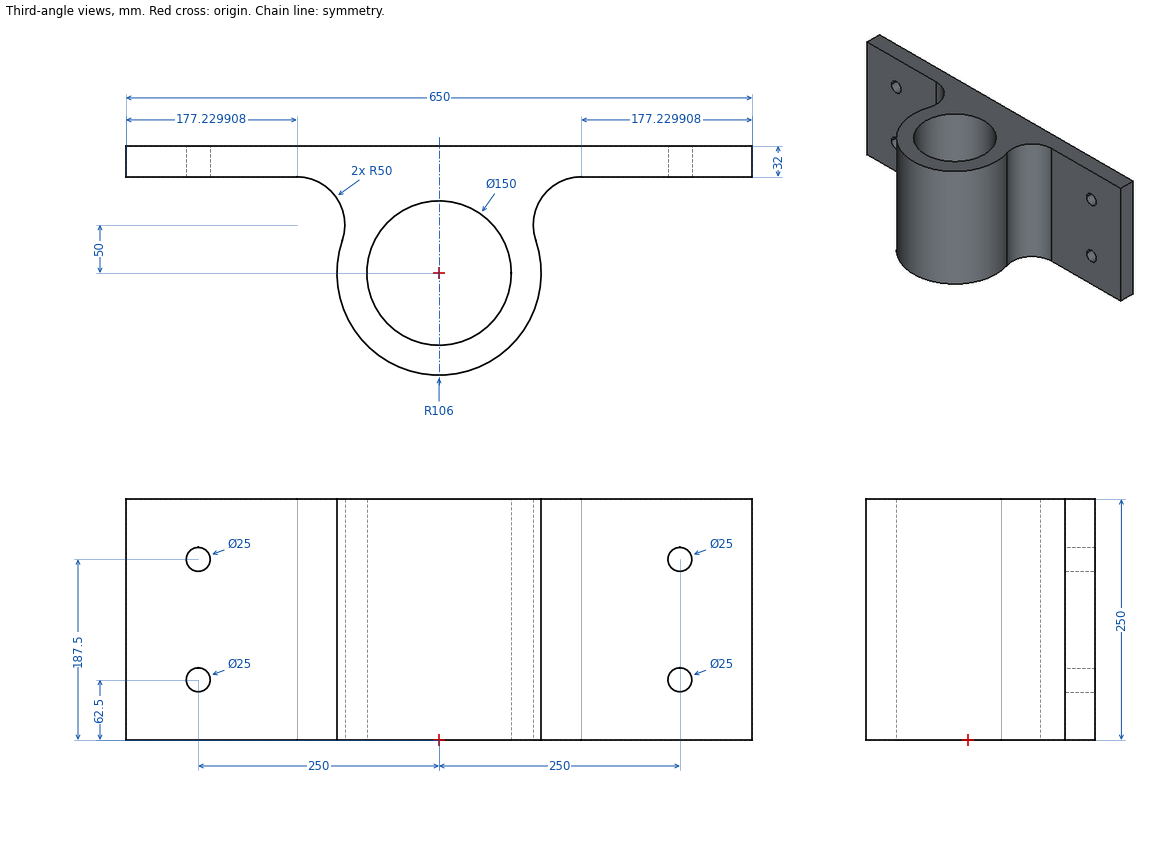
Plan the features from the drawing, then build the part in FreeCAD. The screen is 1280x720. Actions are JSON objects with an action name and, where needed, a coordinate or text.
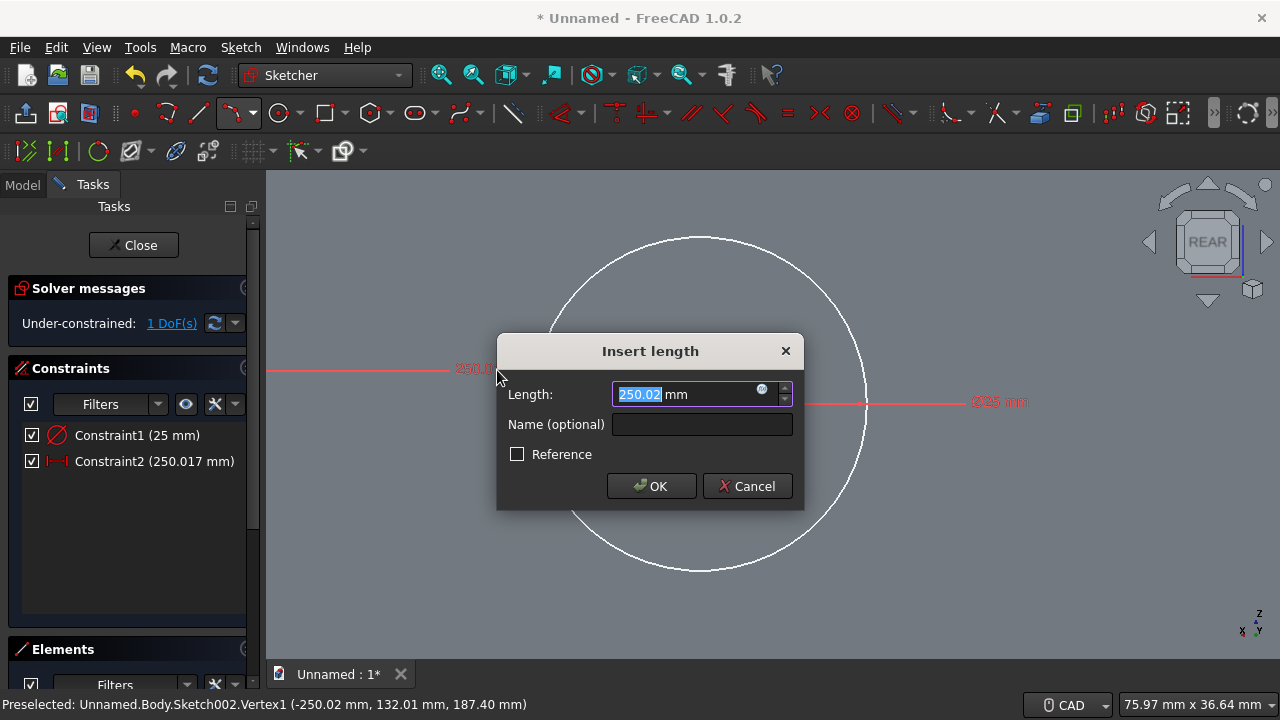
{"action": "type", "text": "250"}
{"action": "key", "text": "Return"}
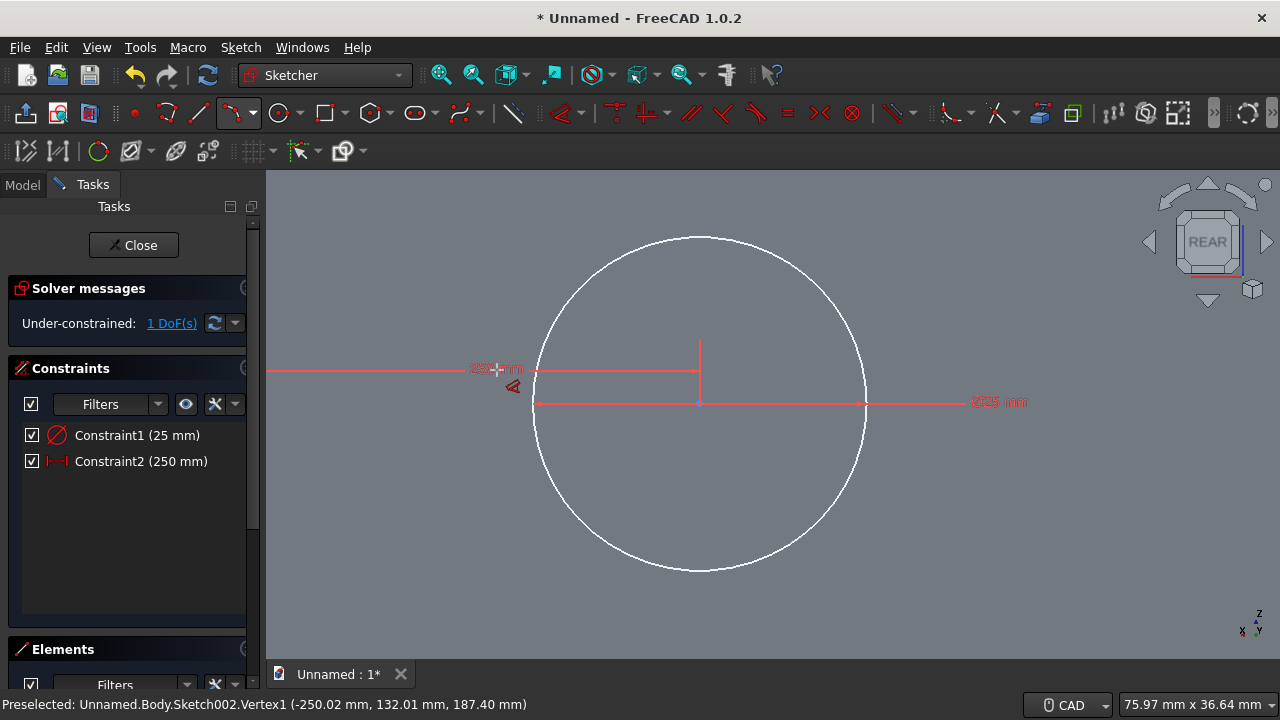
{"action": "left_click", "coordinate": [700, 404]}
{"action": "left_click", "coordinate": [734, 518]}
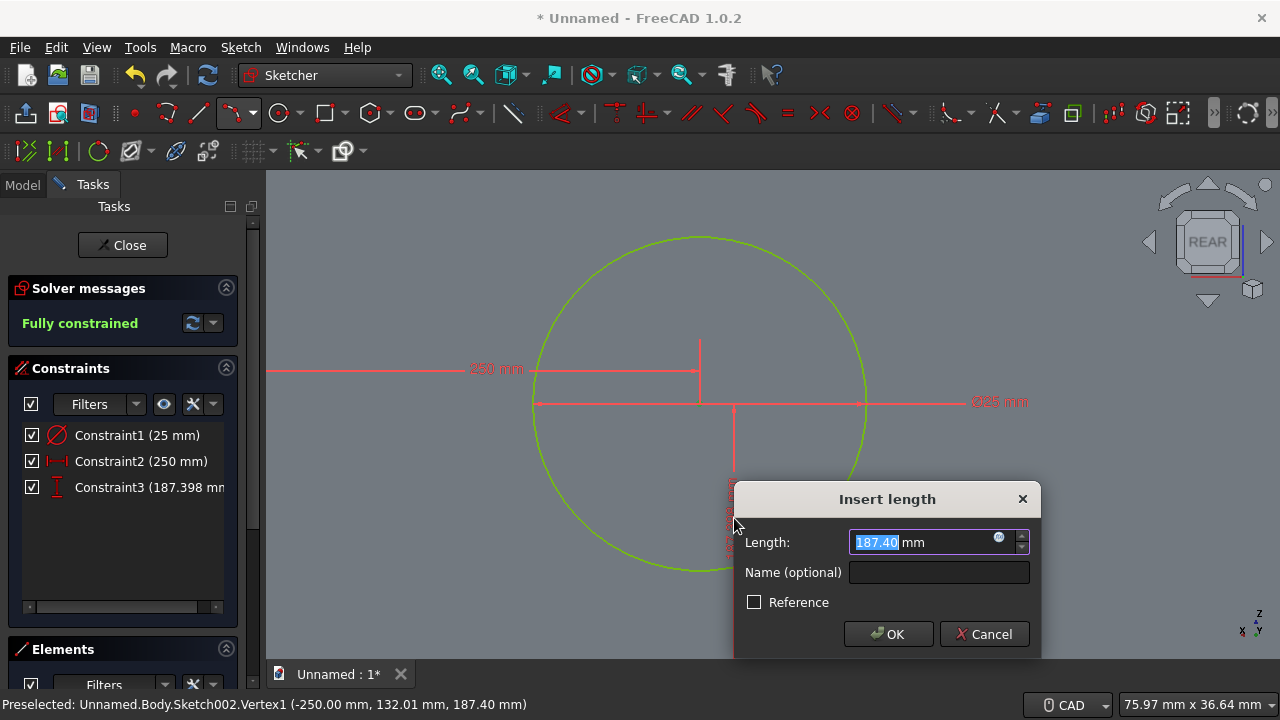
{"action": "type", "text": "187.5"}
{"action": "key", "text": "Return"}
{"action": "key", "text": "Escape"}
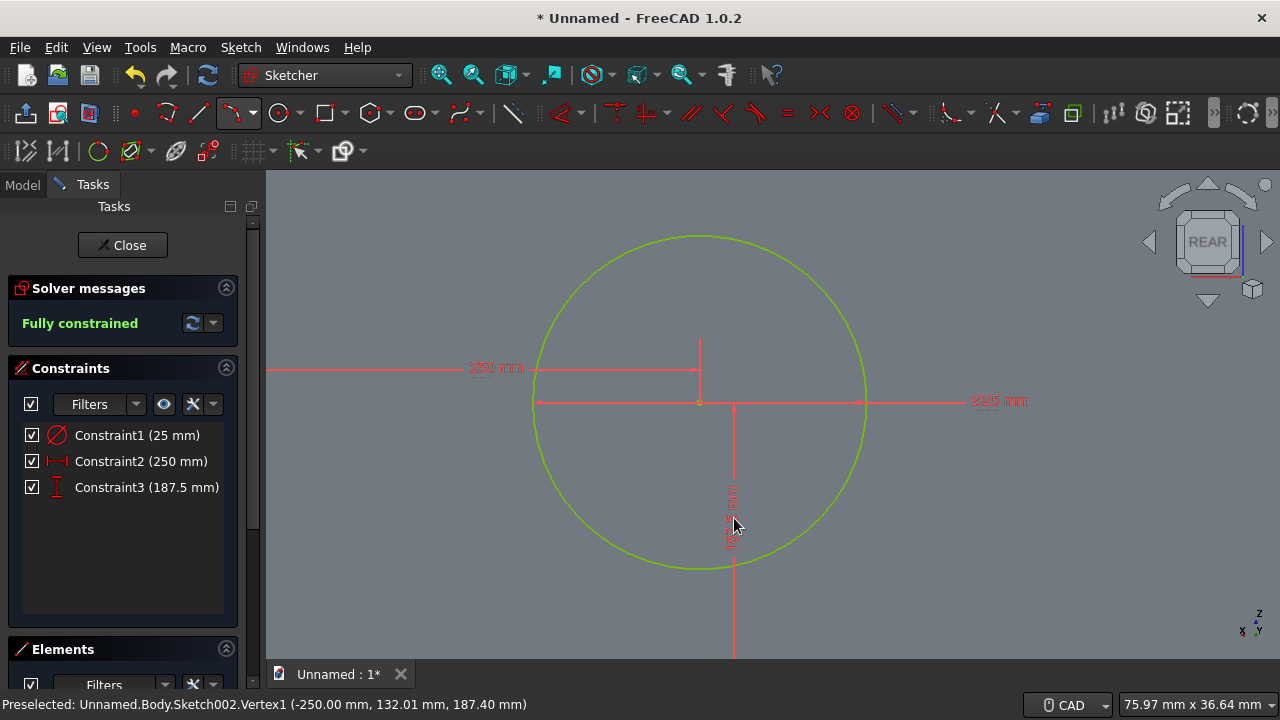
{"action": "left_click", "coordinate": [123, 245]}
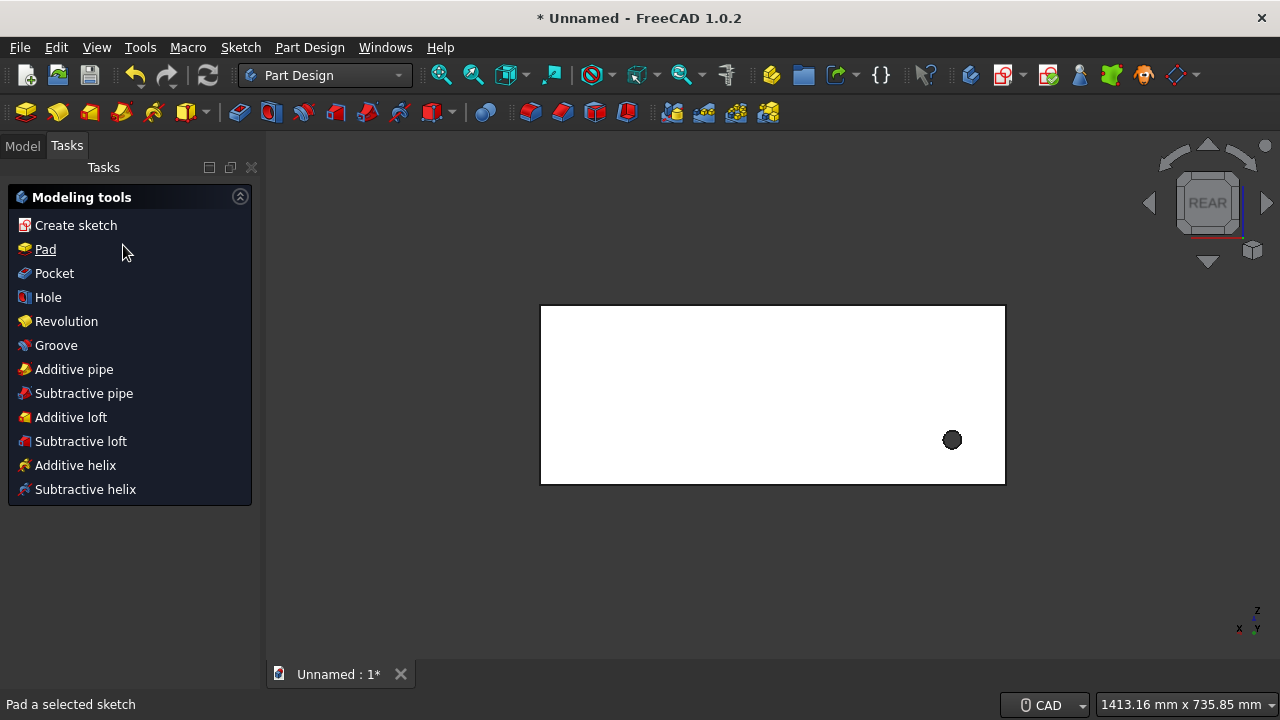
{"action": "left_click", "coordinate": [240, 112]}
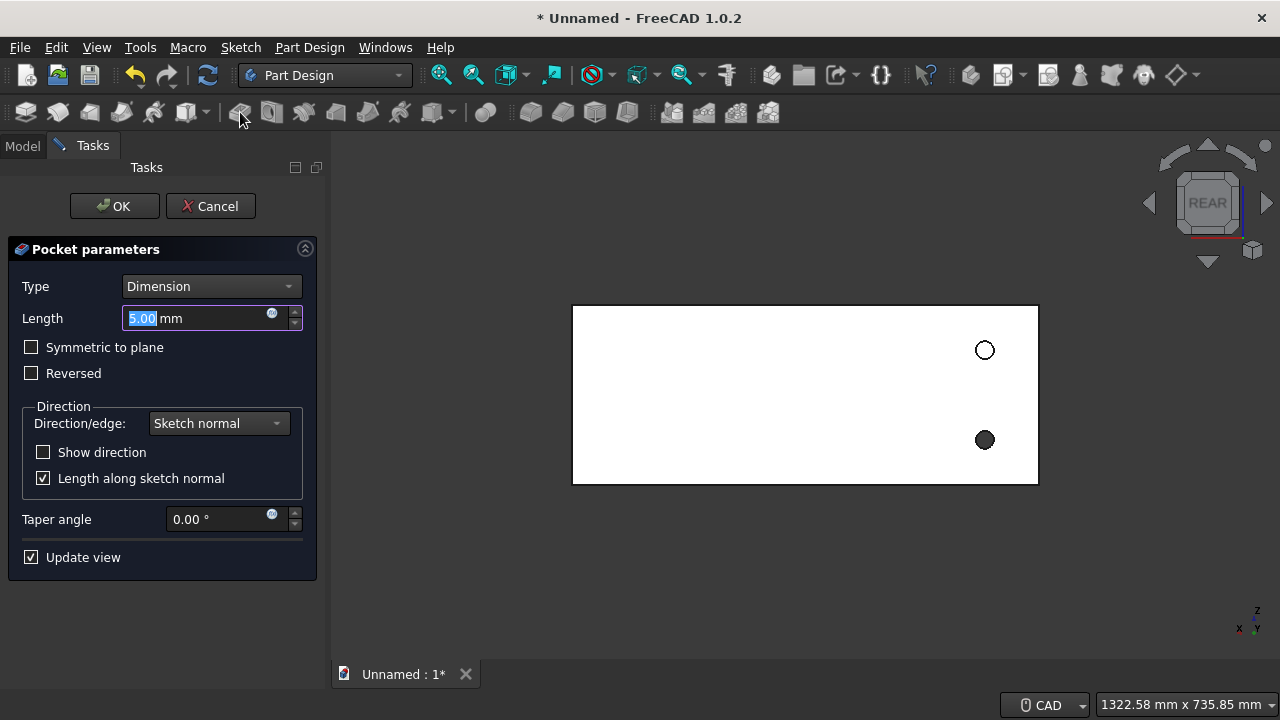
{"action": "left_click", "coordinate": [212, 286]}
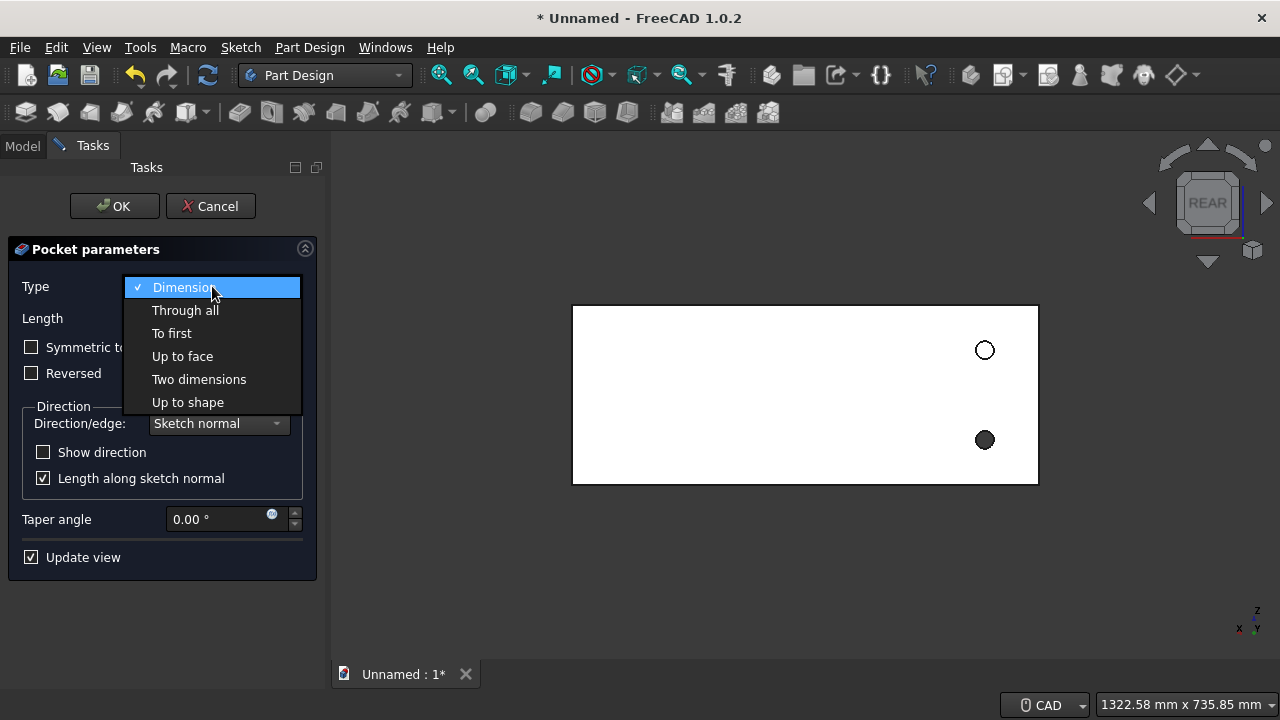
{"action": "left_click", "coordinate": [212, 334]}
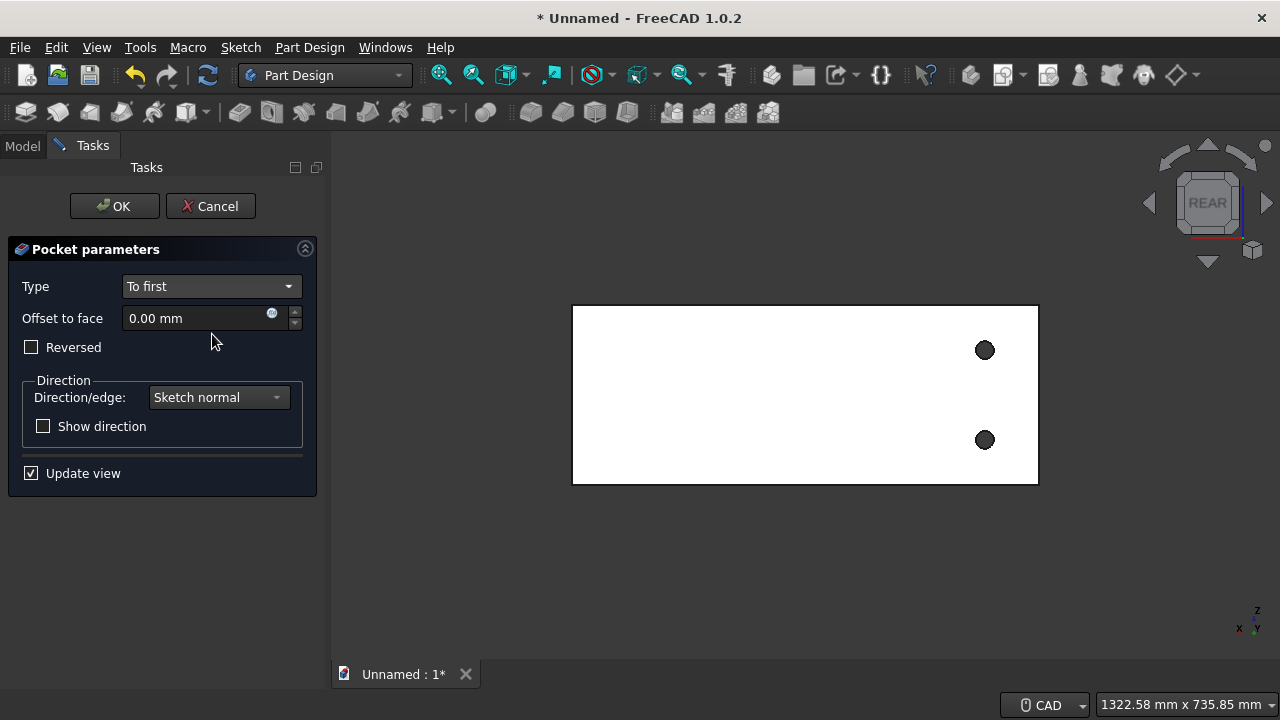
{"action": "left_click", "coordinate": [115, 206]}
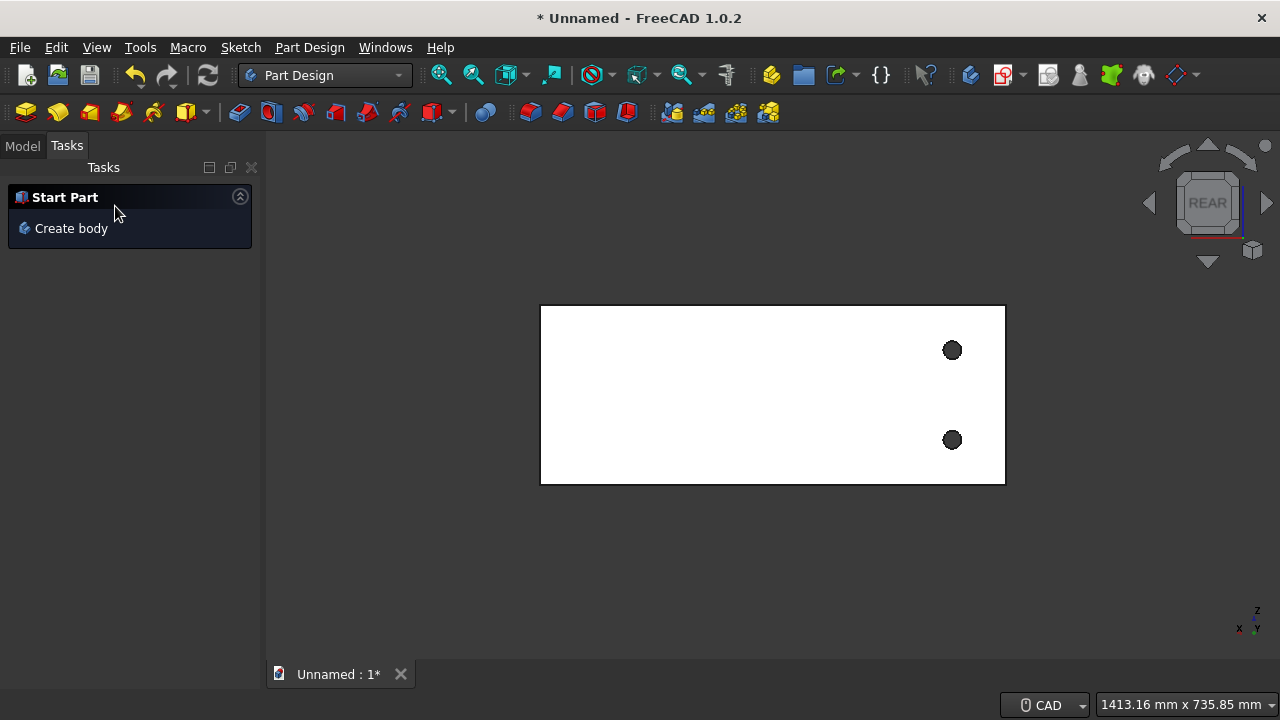
{"action": "left_click", "coordinate": [640, 394]}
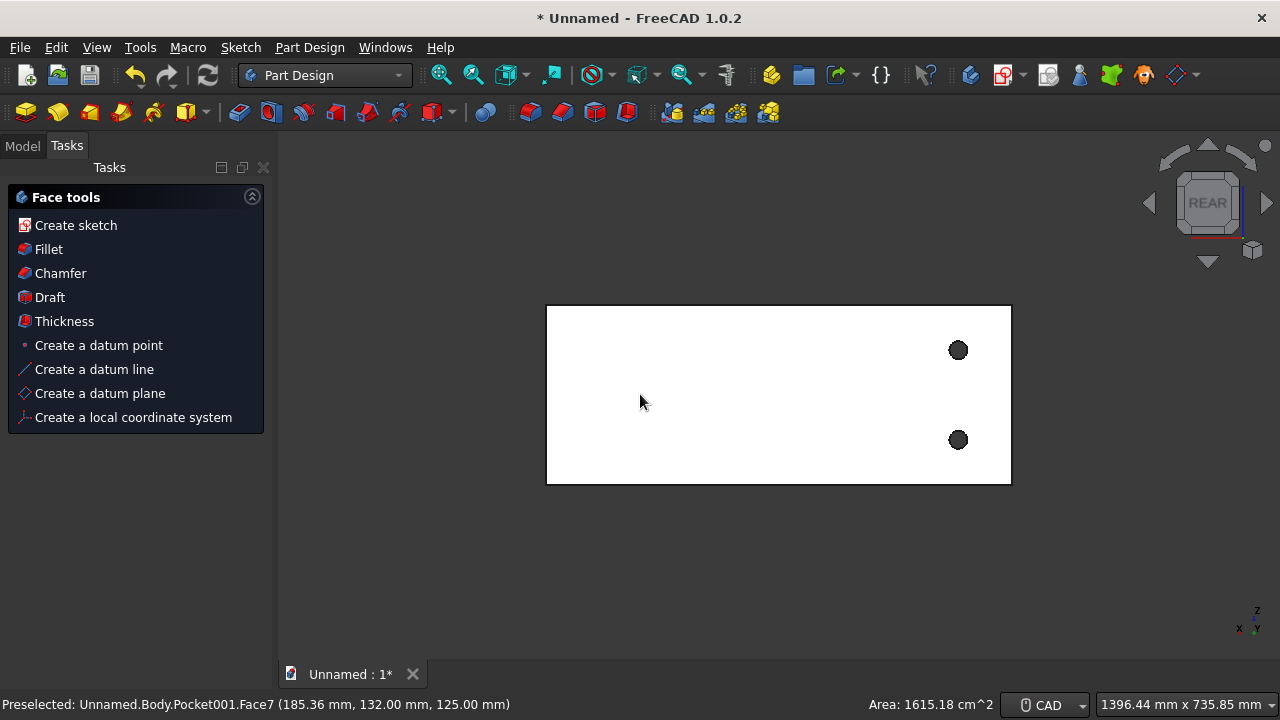
{"action": "left_click", "coordinate": [1004, 76]}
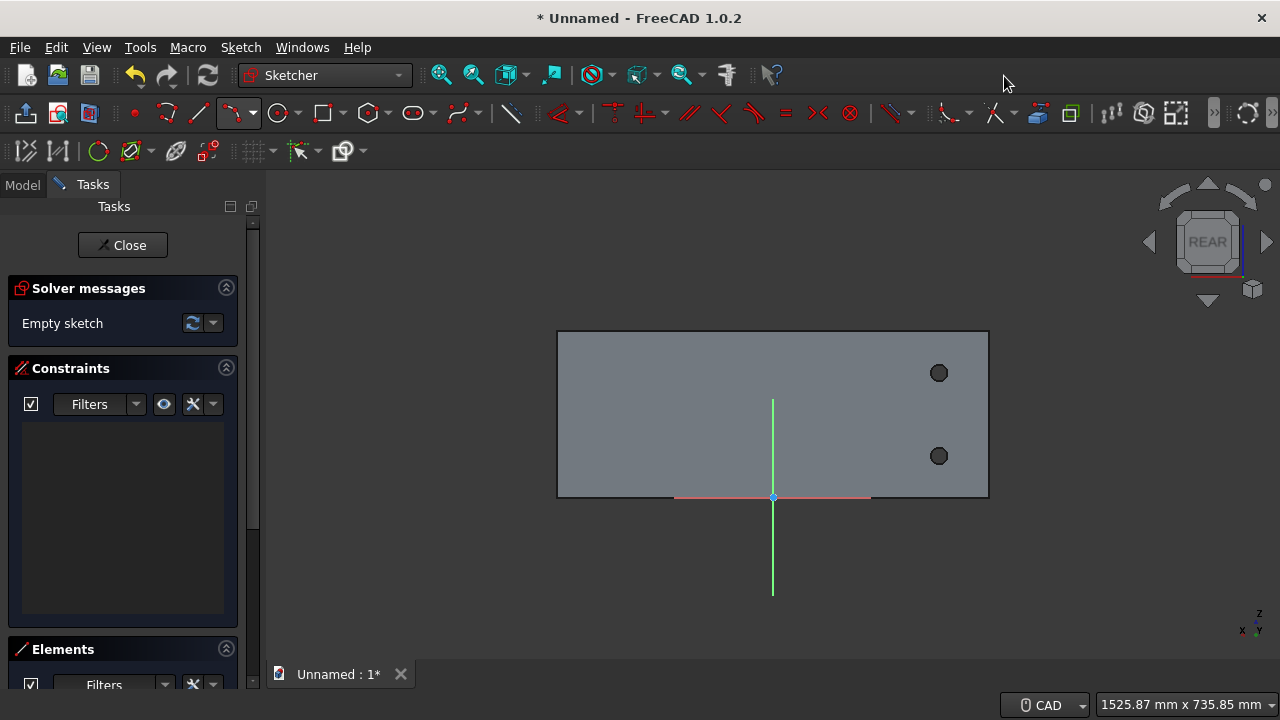
{"action": "scroll", "coordinate": [602, 371], "scroll_direction": "up", "scroll_amount": 15}